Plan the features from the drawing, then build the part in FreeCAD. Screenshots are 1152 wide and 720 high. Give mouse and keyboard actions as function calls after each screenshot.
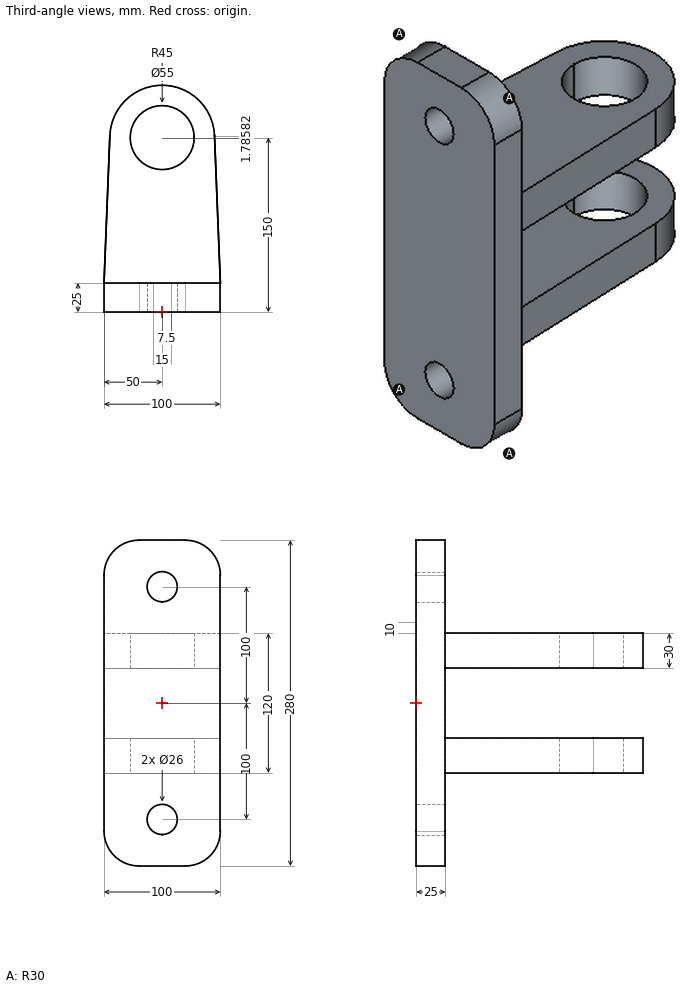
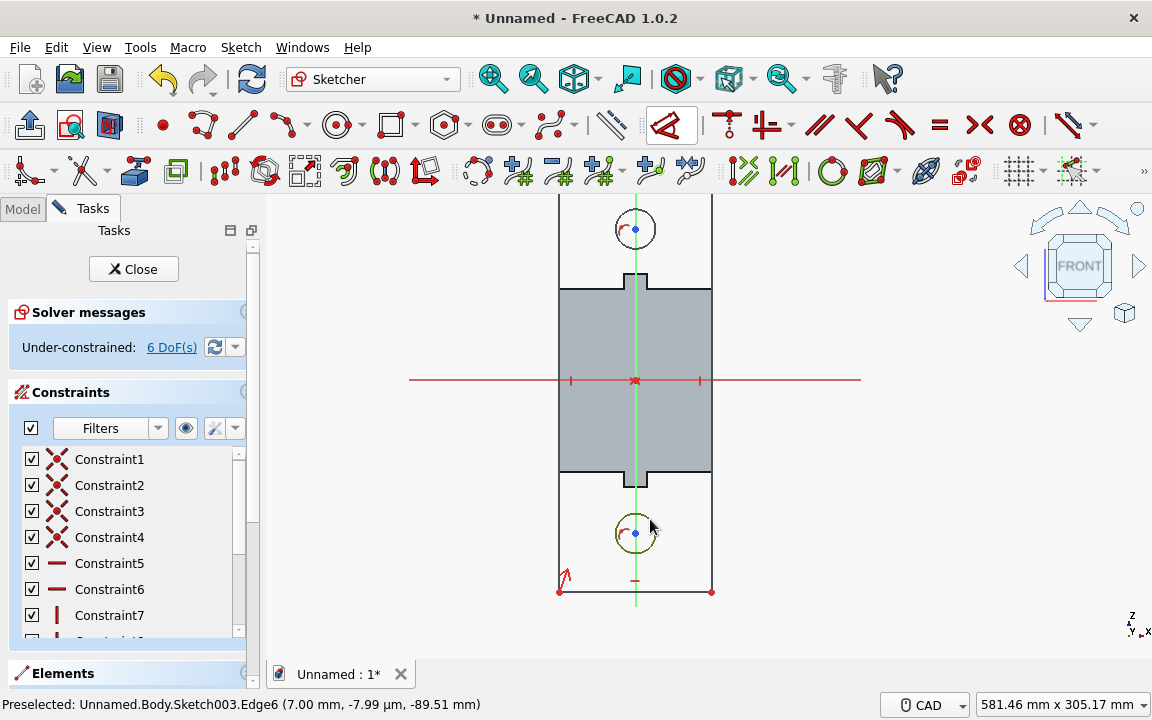
click(622, 243)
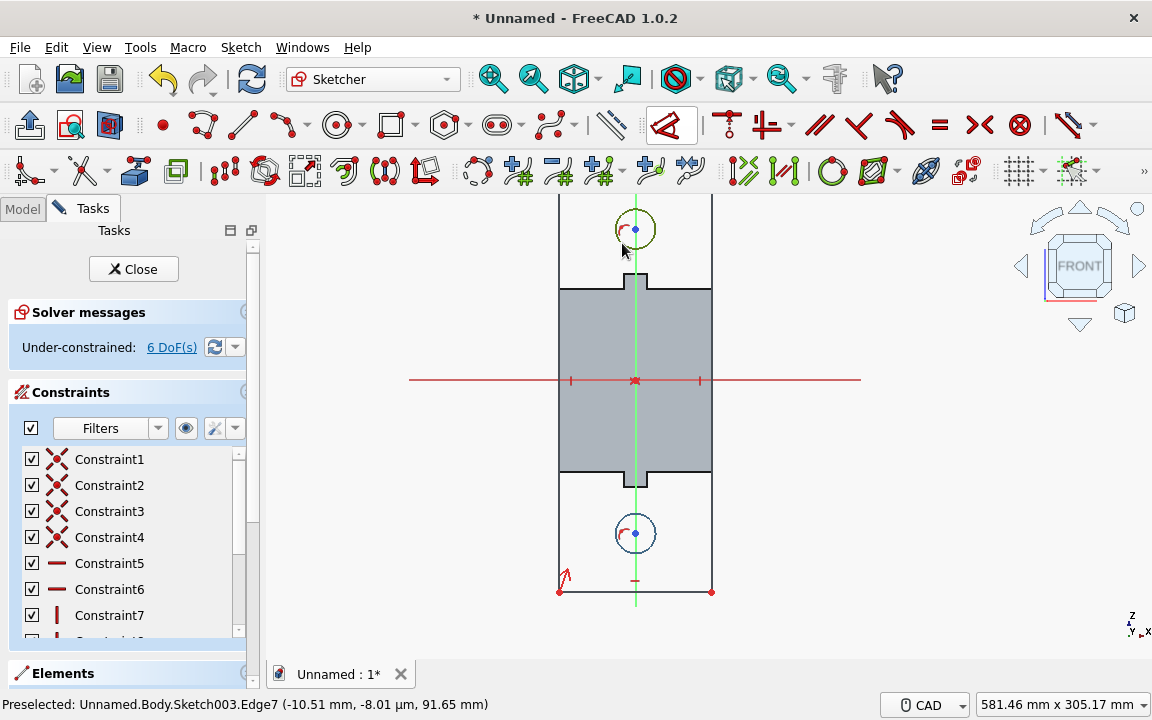
click(940, 126)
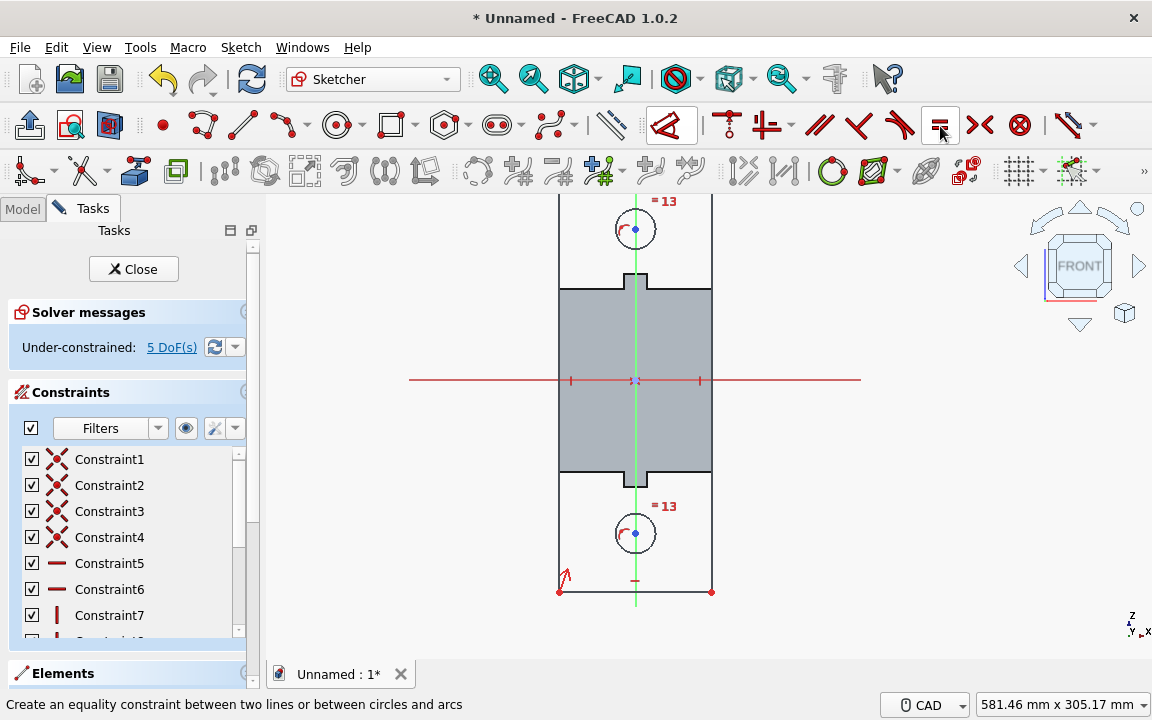
click(650, 519)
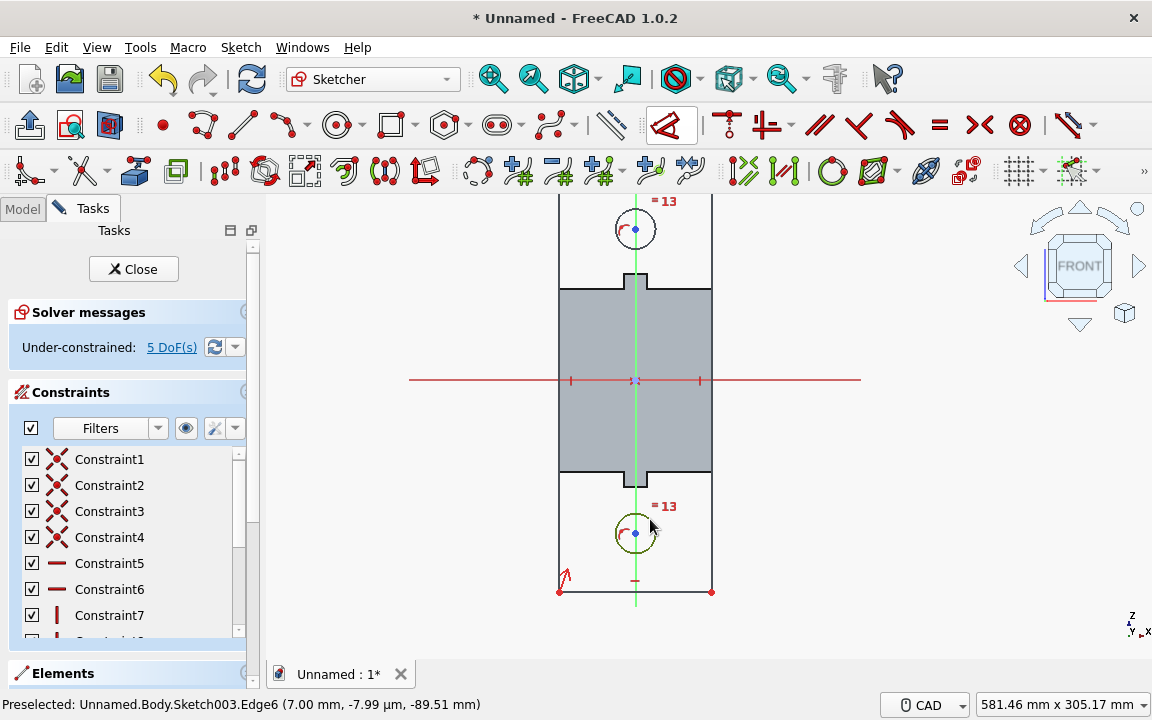
key(k)
key(o)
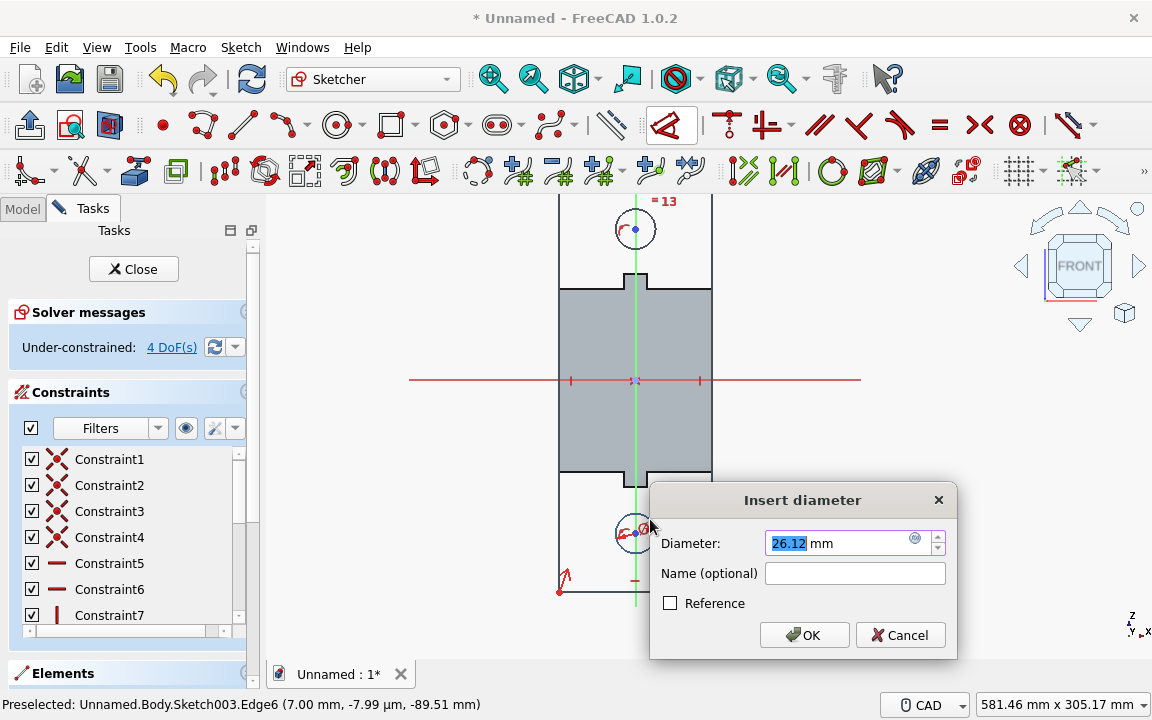
text(26)
key(Return)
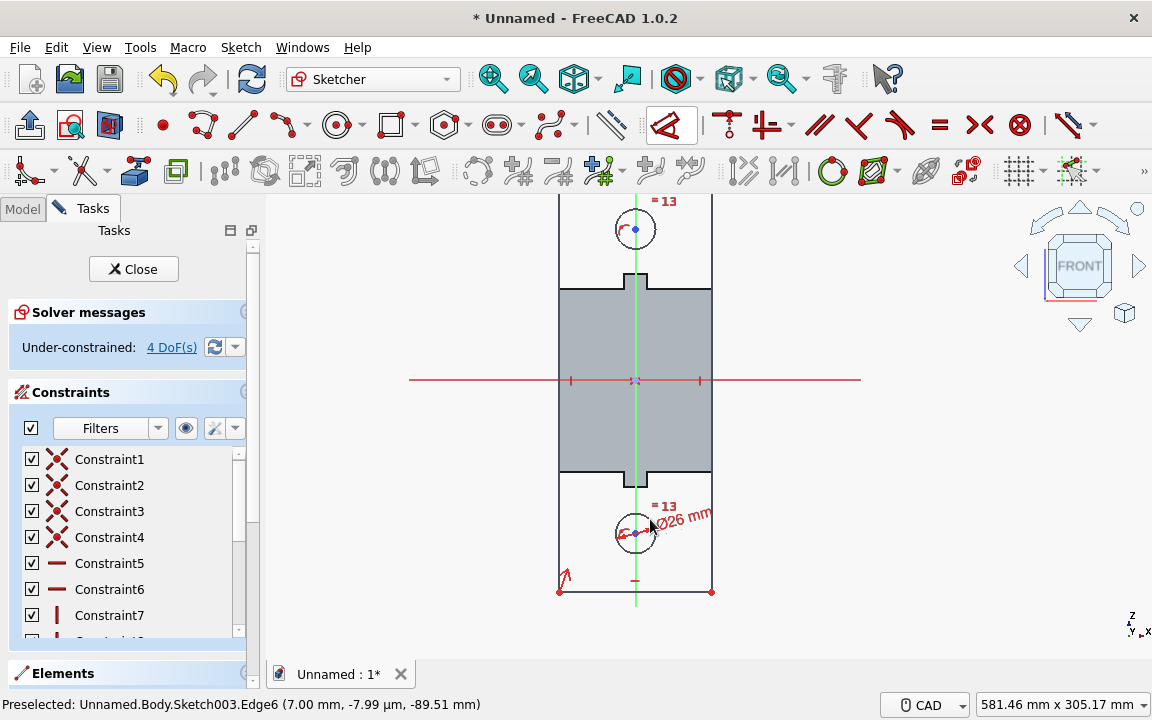
click(605, 592)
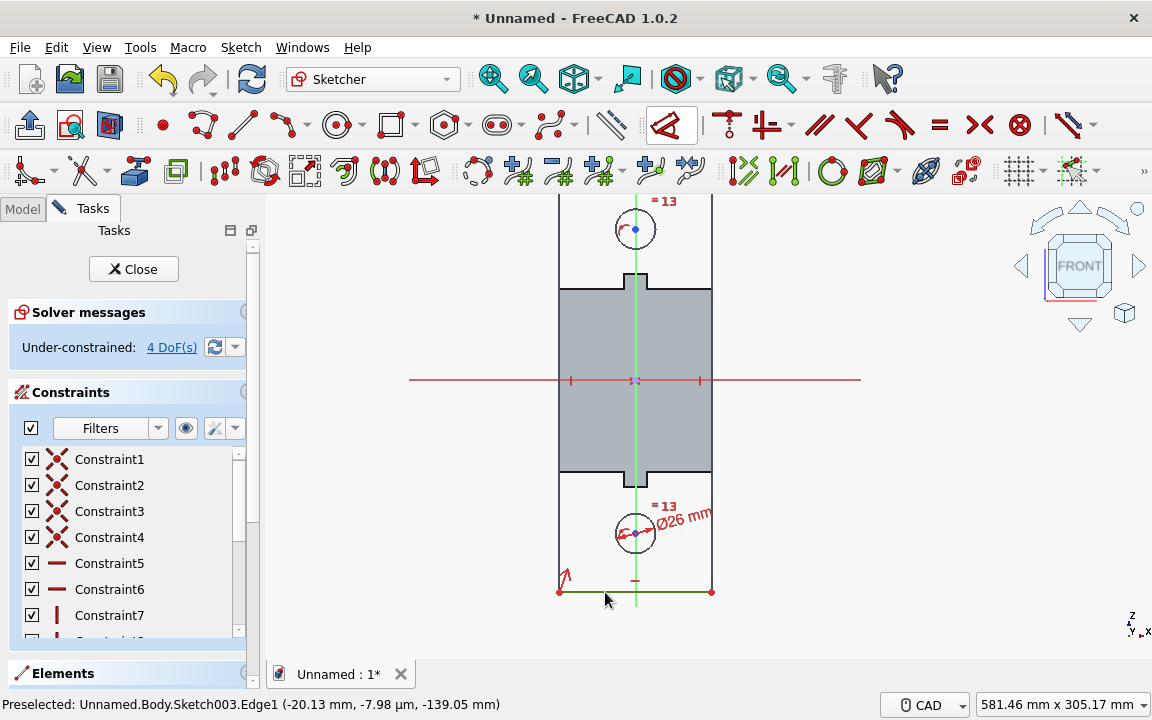
click(692, 126)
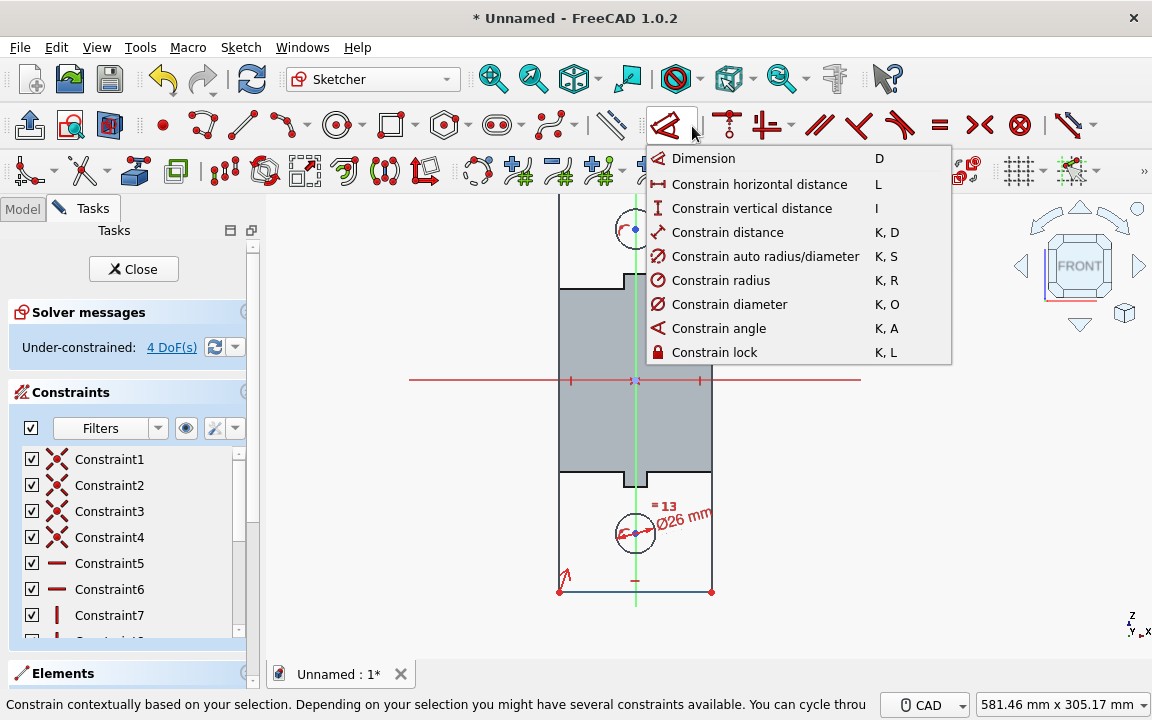
click(799, 184)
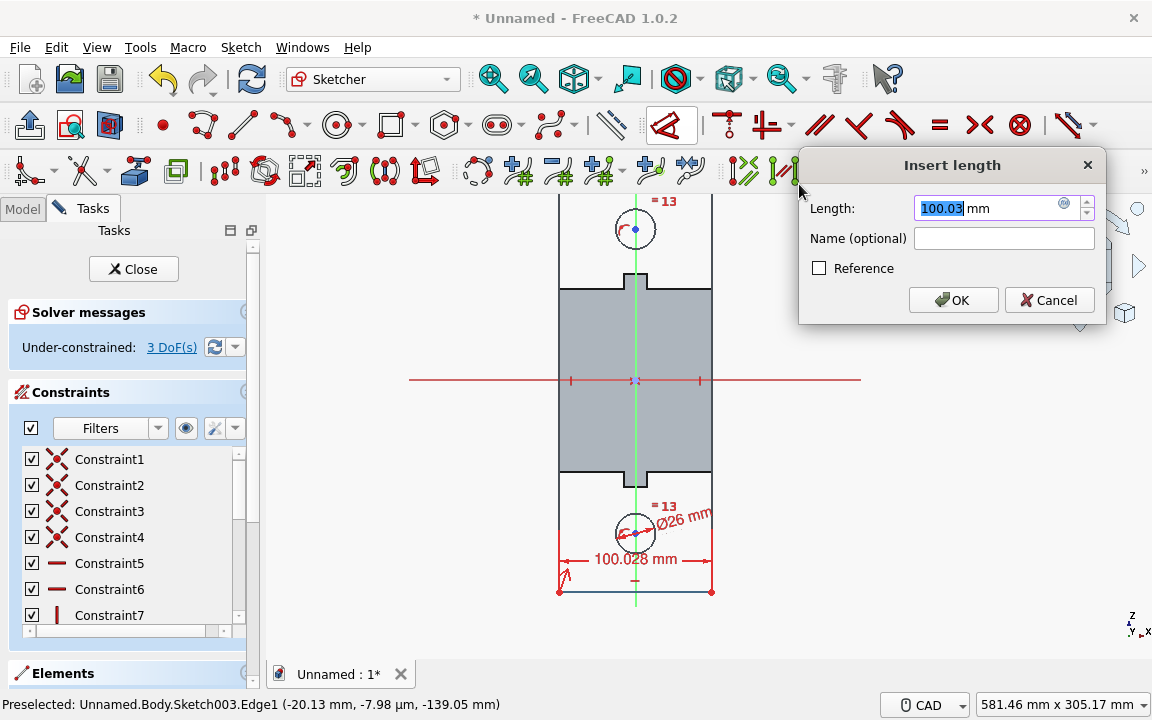
text(100)
key(Return)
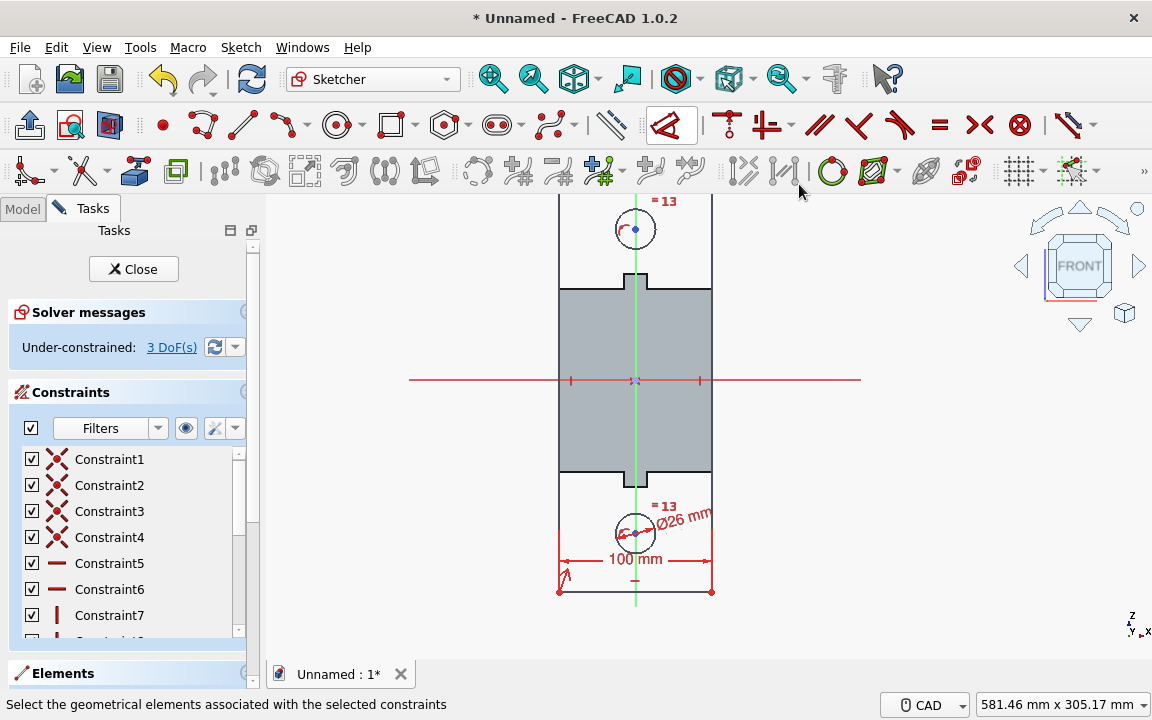
click(712, 465)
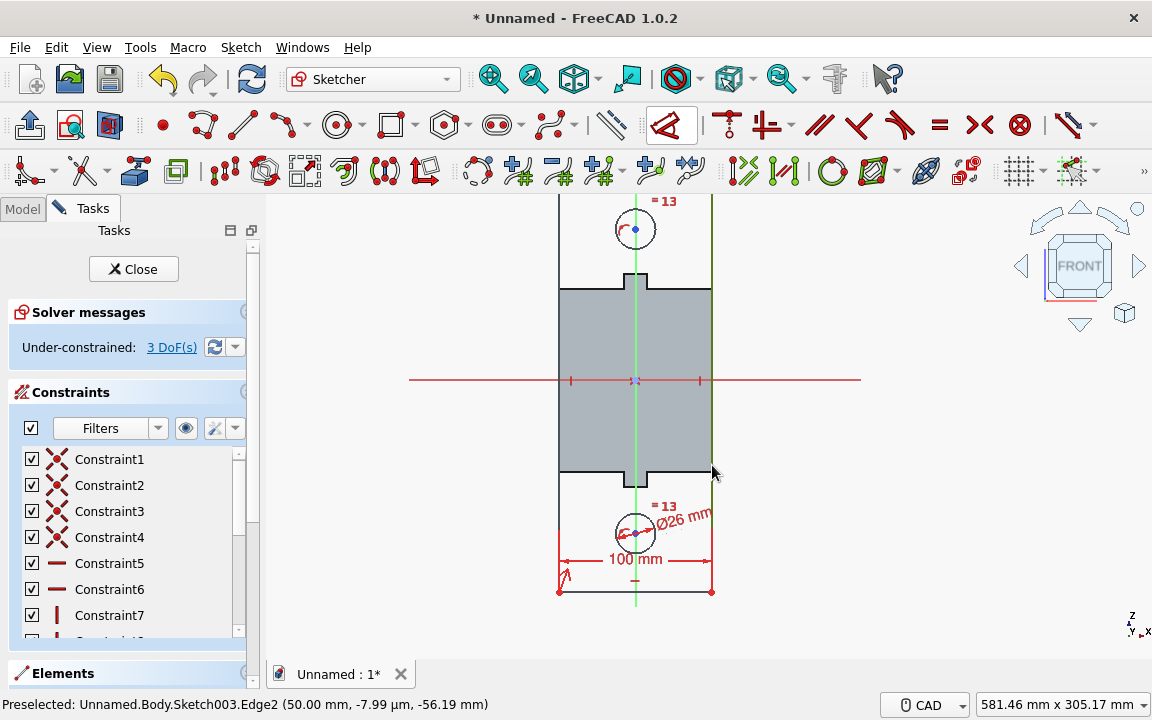
click(692, 126)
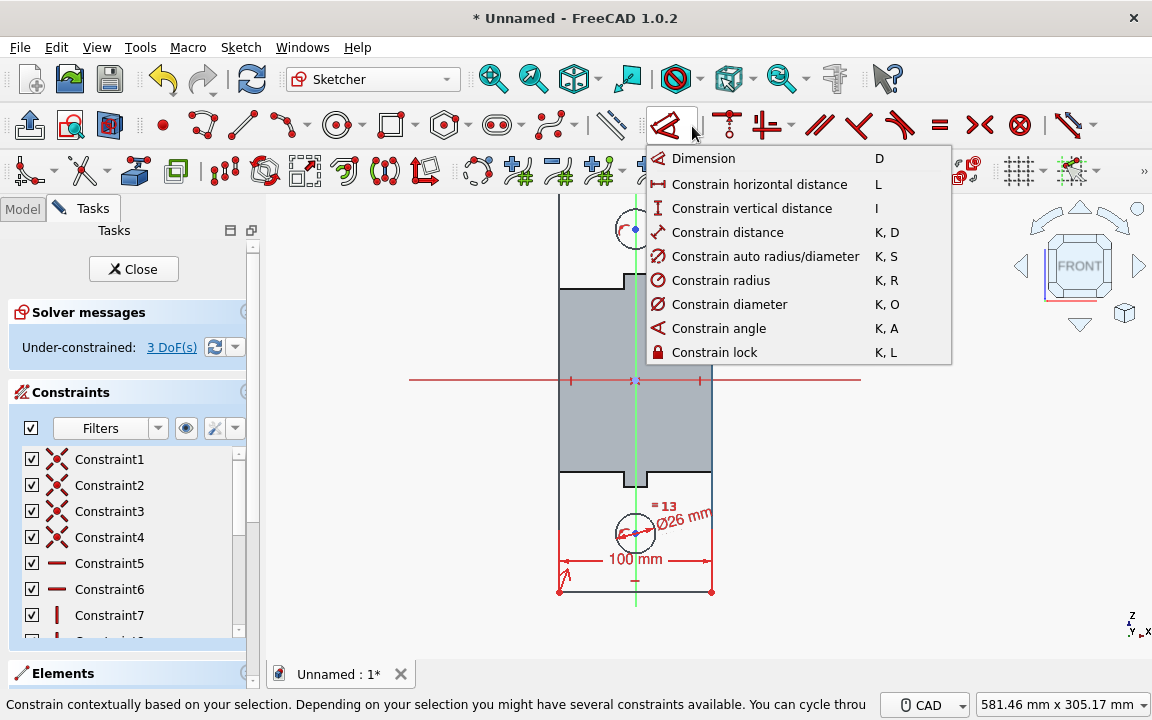
click(799, 208)